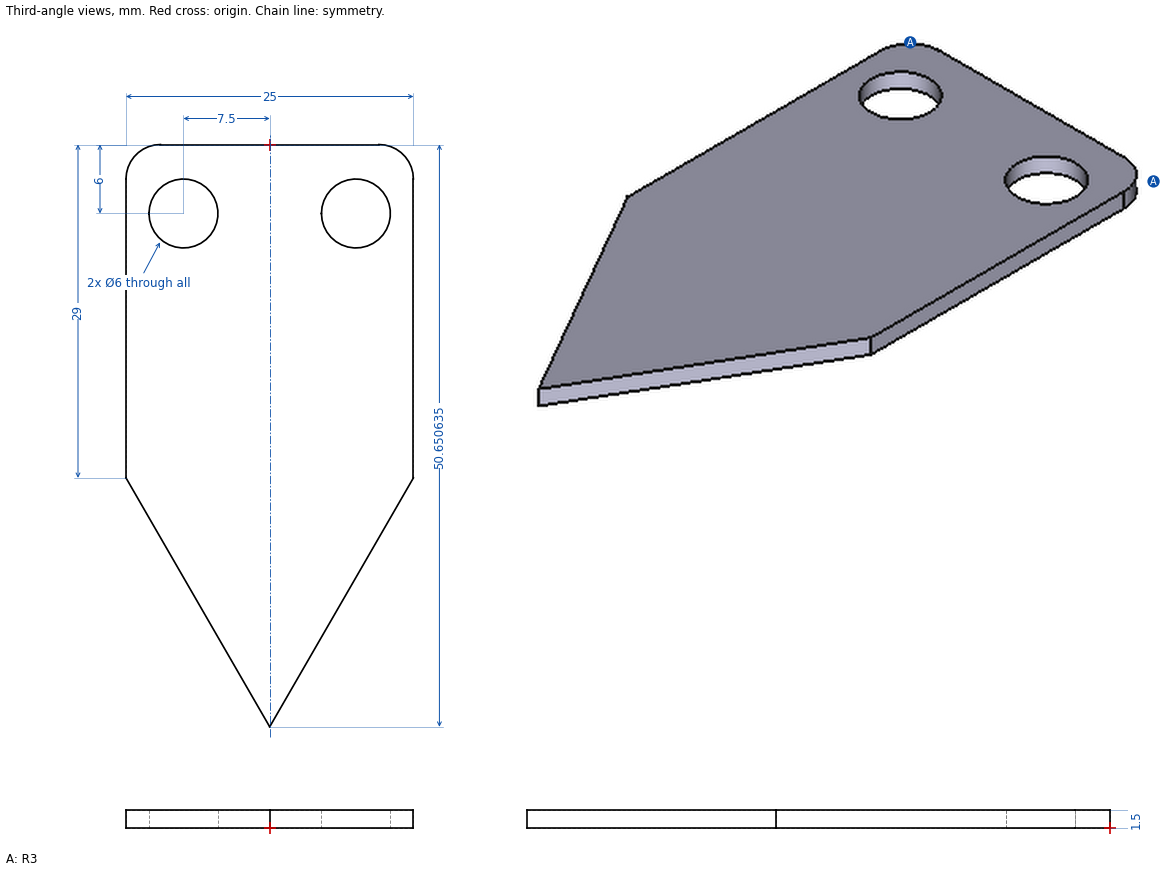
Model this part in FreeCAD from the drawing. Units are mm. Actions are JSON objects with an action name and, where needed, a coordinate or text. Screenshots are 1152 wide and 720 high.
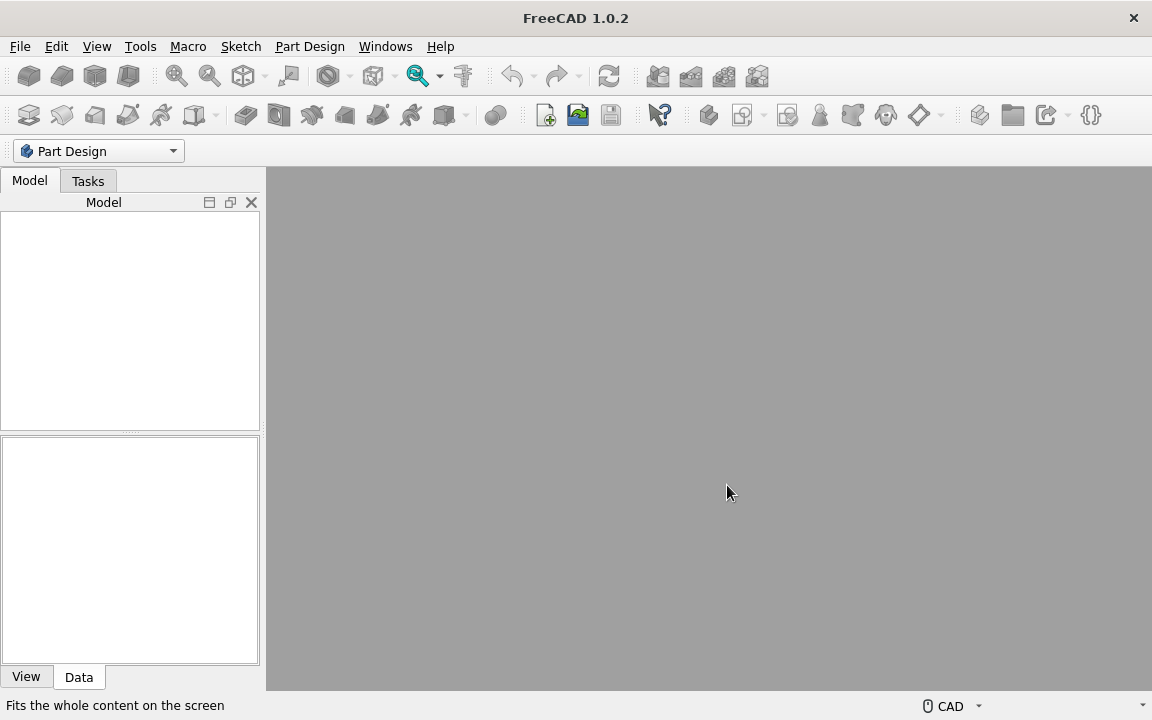
{"action": "left_click", "coordinate": [545, 116]}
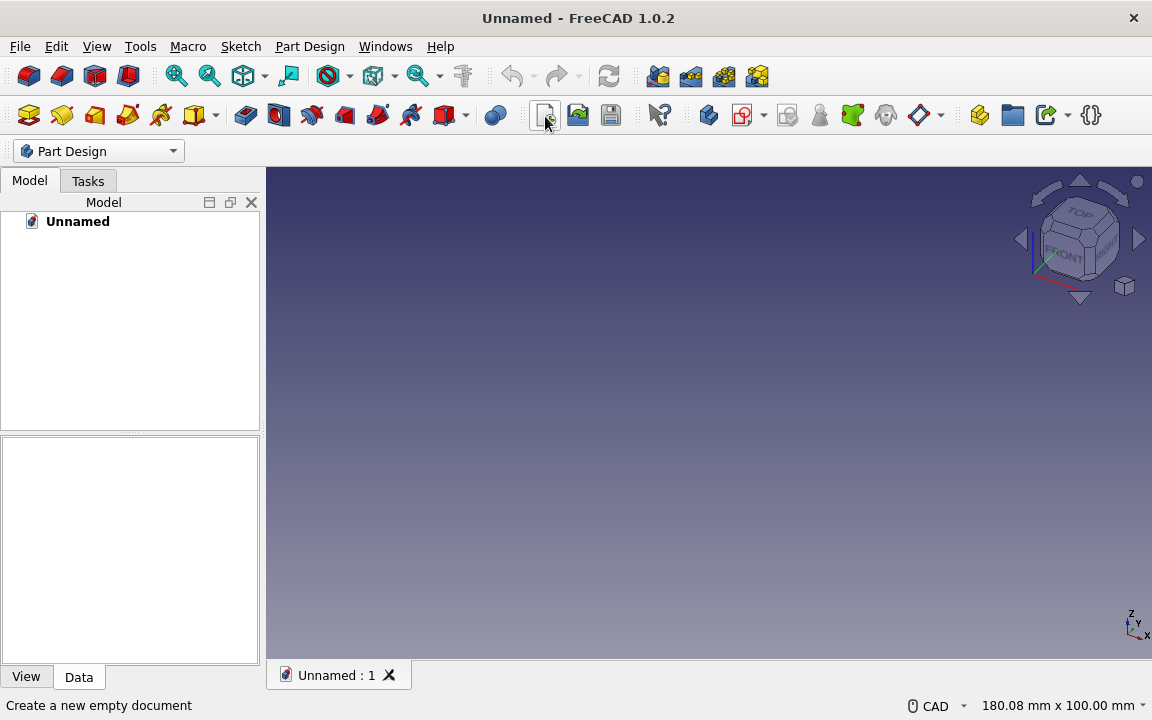
{"action": "left_click", "coordinate": [742, 116]}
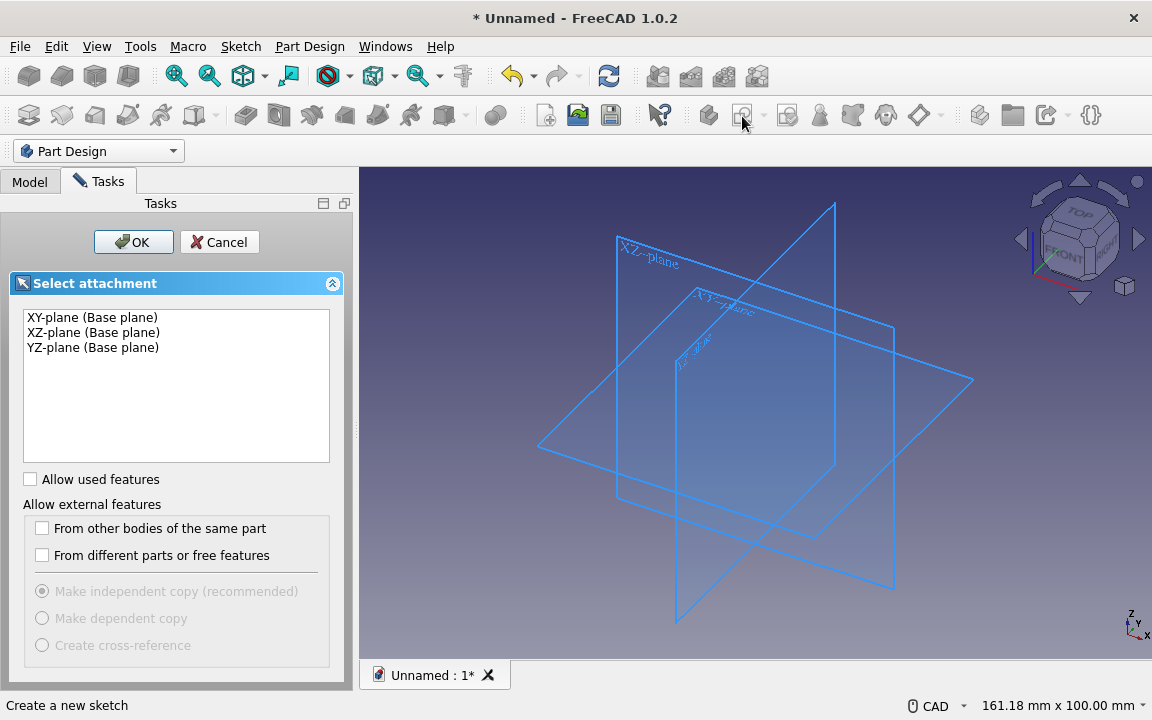
{"action": "left_click", "coordinate": [84, 318]}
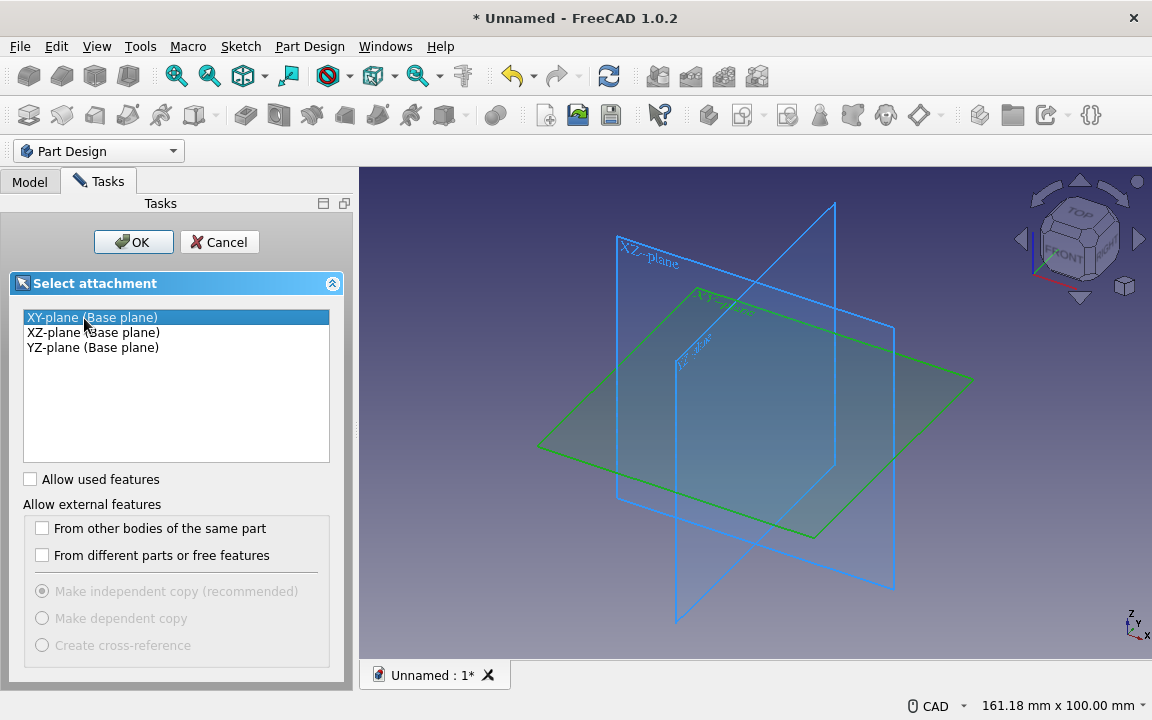
{"action": "left_click", "coordinate": [134, 242]}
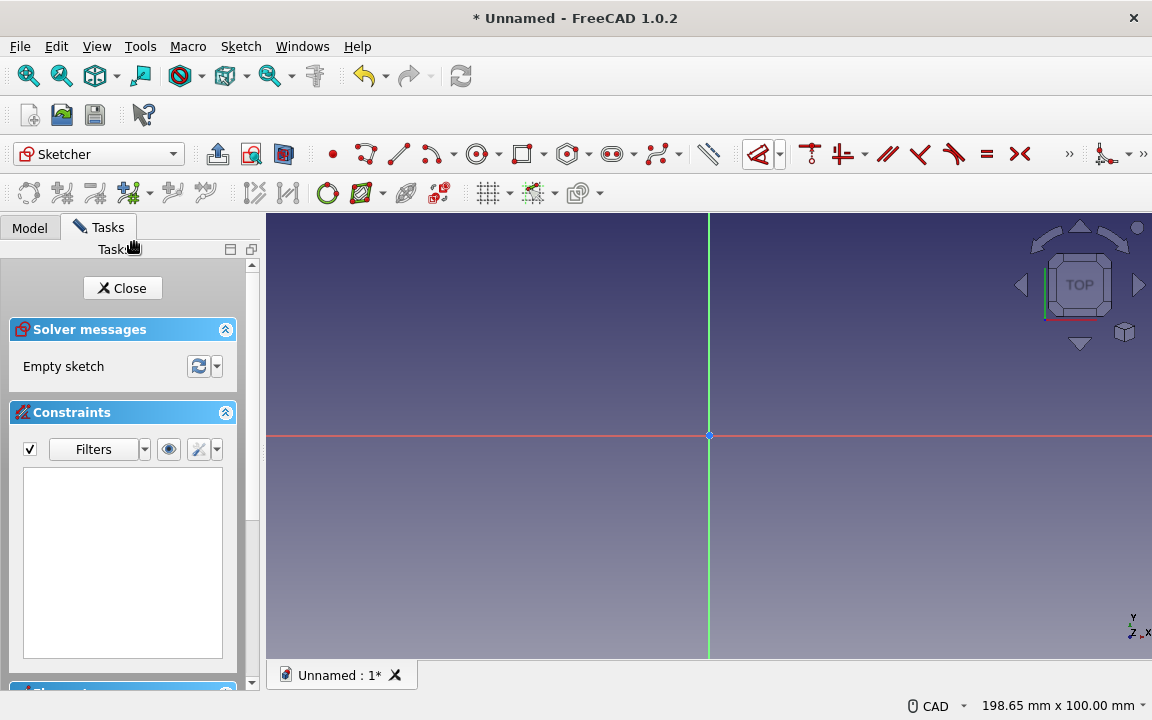
{"action": "scroll", "coordinate": [331, 241], "scroll_direction": "down", "scroll_amount": 1}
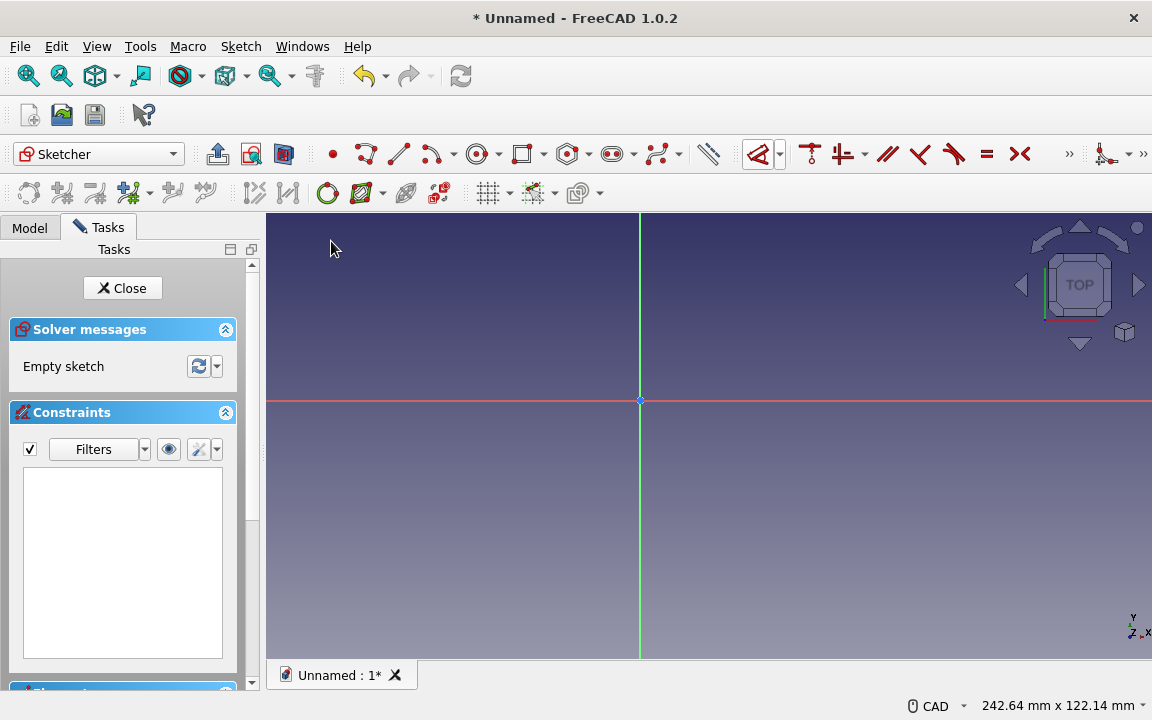
{"action": "scroll", "coordinate": [640, 609], "scroll_direction": "up", "scroll_amount": 2}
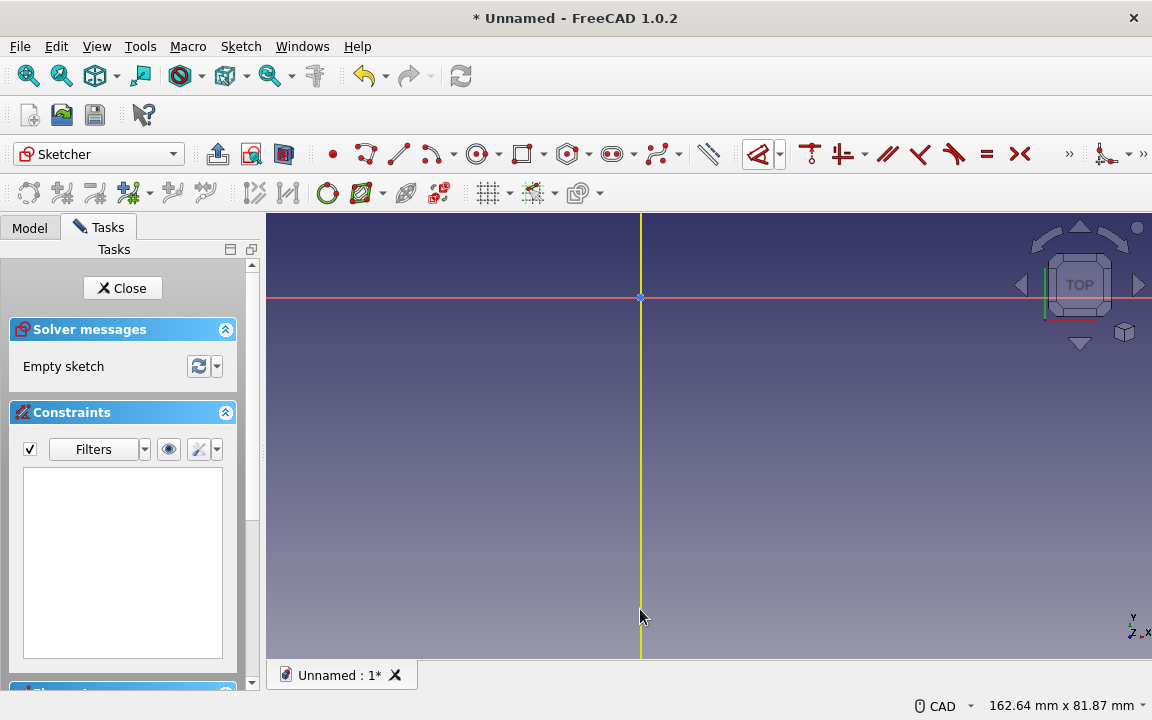
{"action": "left_click", "coordinate": [366, 154]}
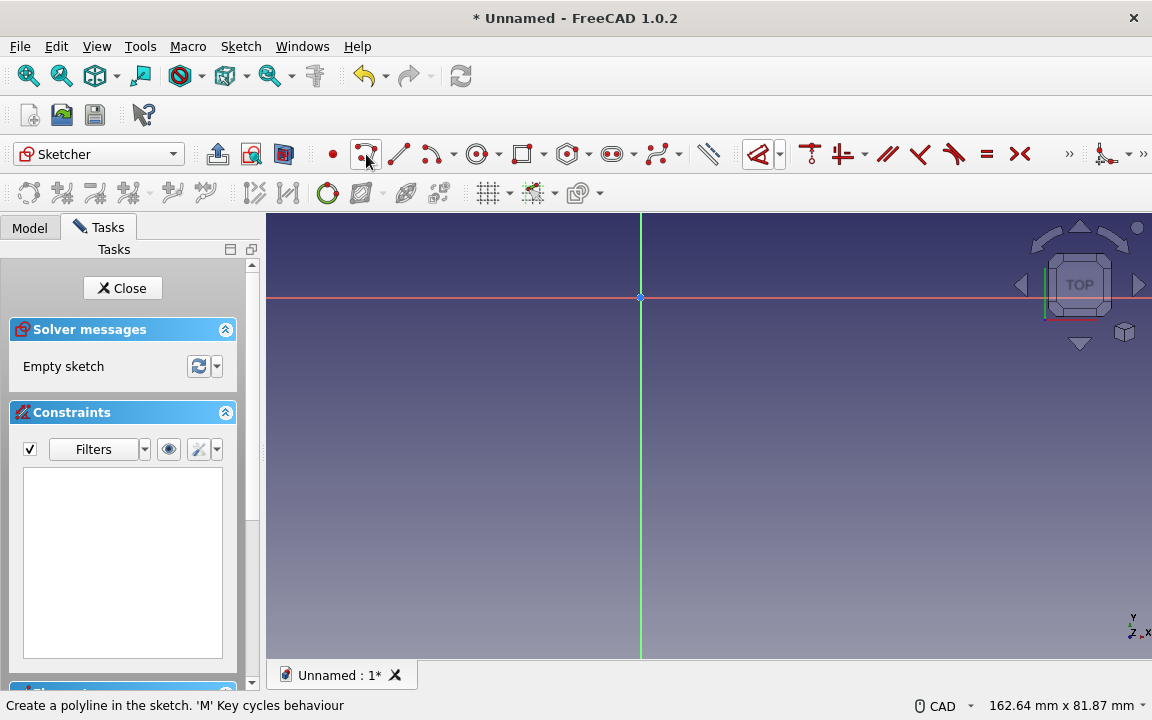
{"action": "left_click", "coordinate": [709, 298]}
{"action": "left_click", "coordinate": [572, 307]}
{"action": "left_click", "coordinate": [572, 456]}
{"action": "left_click", "coordinate": [641, 574]}
{"action": "left_click", "coordinate": [709, 456]}
{"action": "left_click", "coordinate": [709, 298]}
{"action": "key", "text": "Escape"}
{"action": "key", "text": "Escape"}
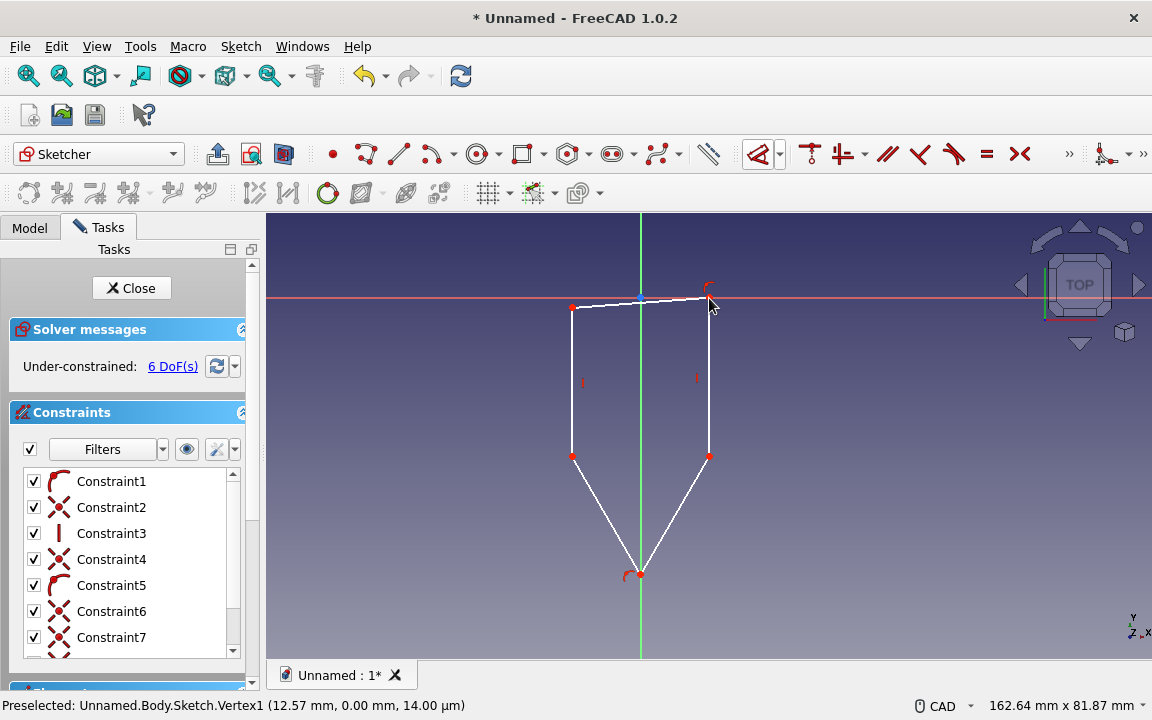
{"action": "left_click", "coordinate": [668, 301]}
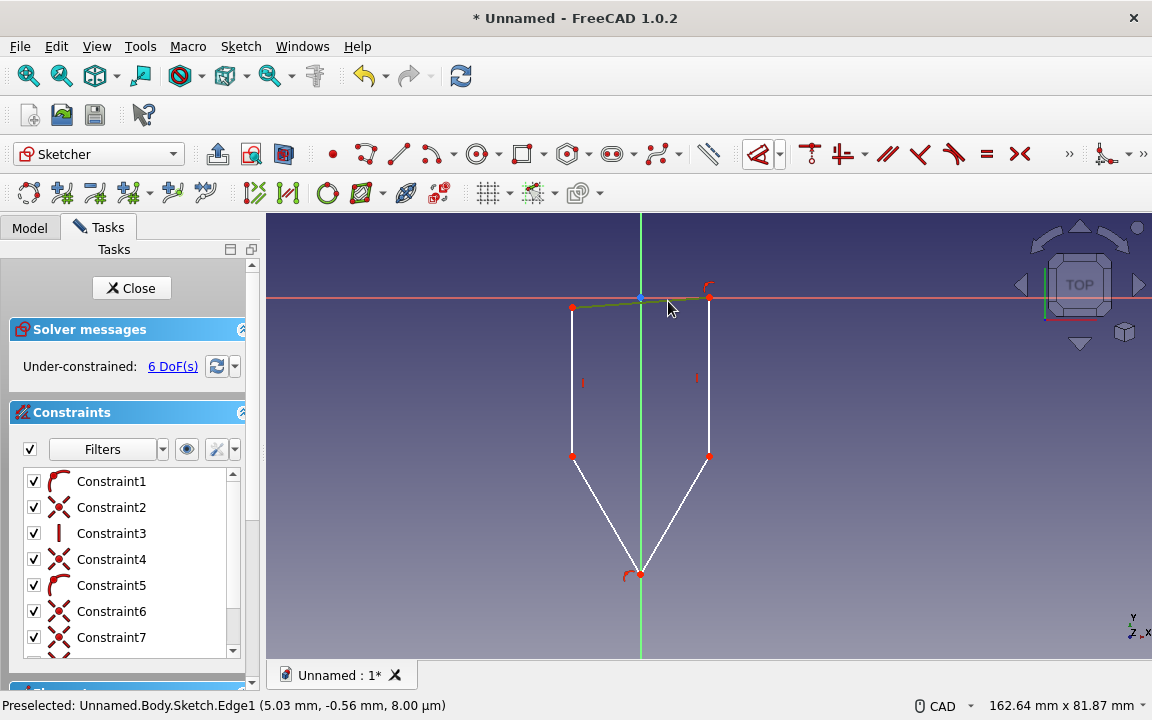
{"action": "key", "text": "h"}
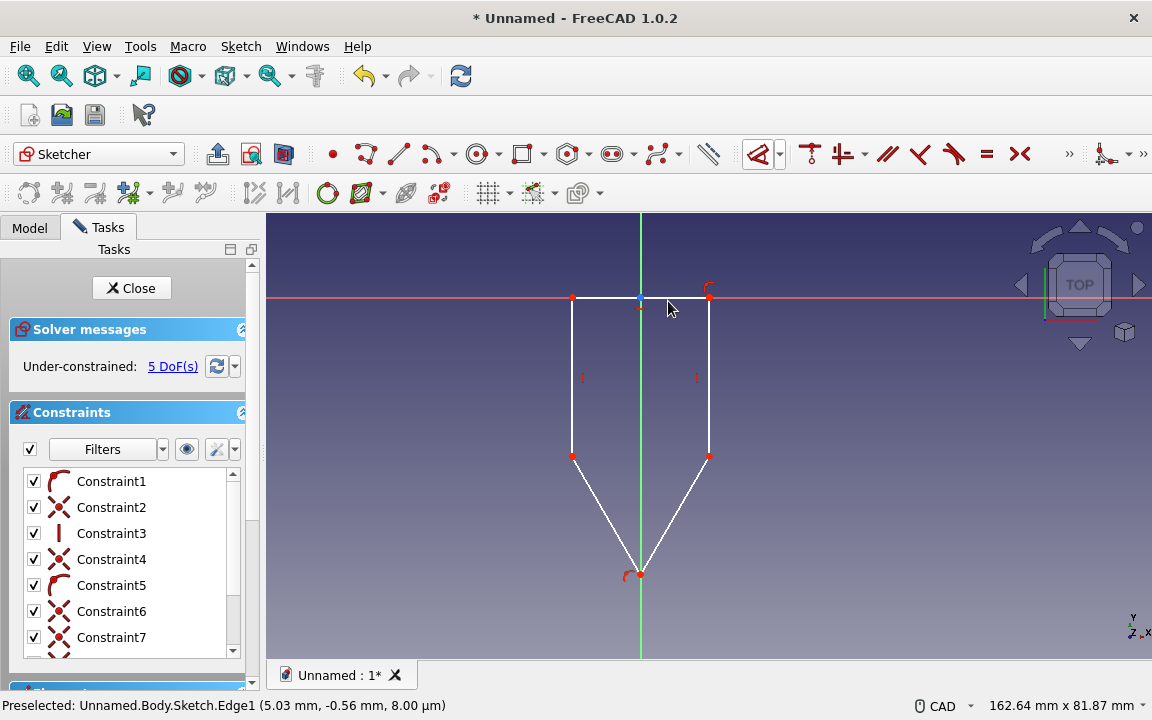
{"action": "left_click", "coordinate": [572, 457]}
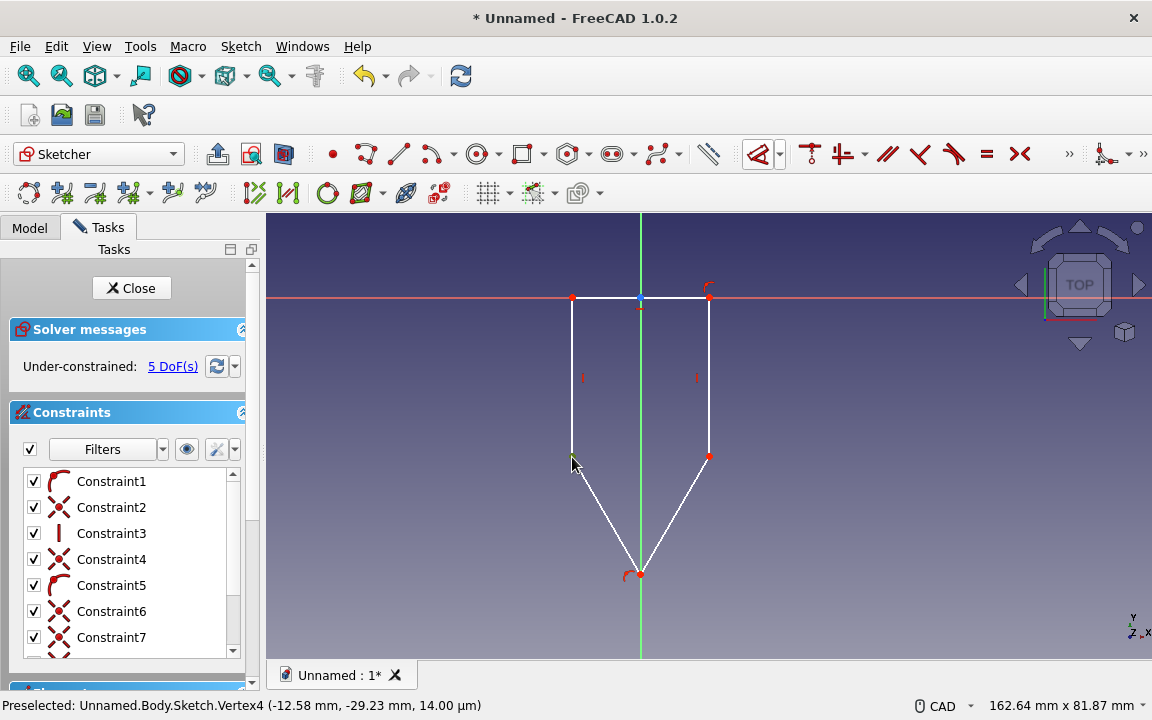
{"action": "left_click", "coordinate": [709, 457]}